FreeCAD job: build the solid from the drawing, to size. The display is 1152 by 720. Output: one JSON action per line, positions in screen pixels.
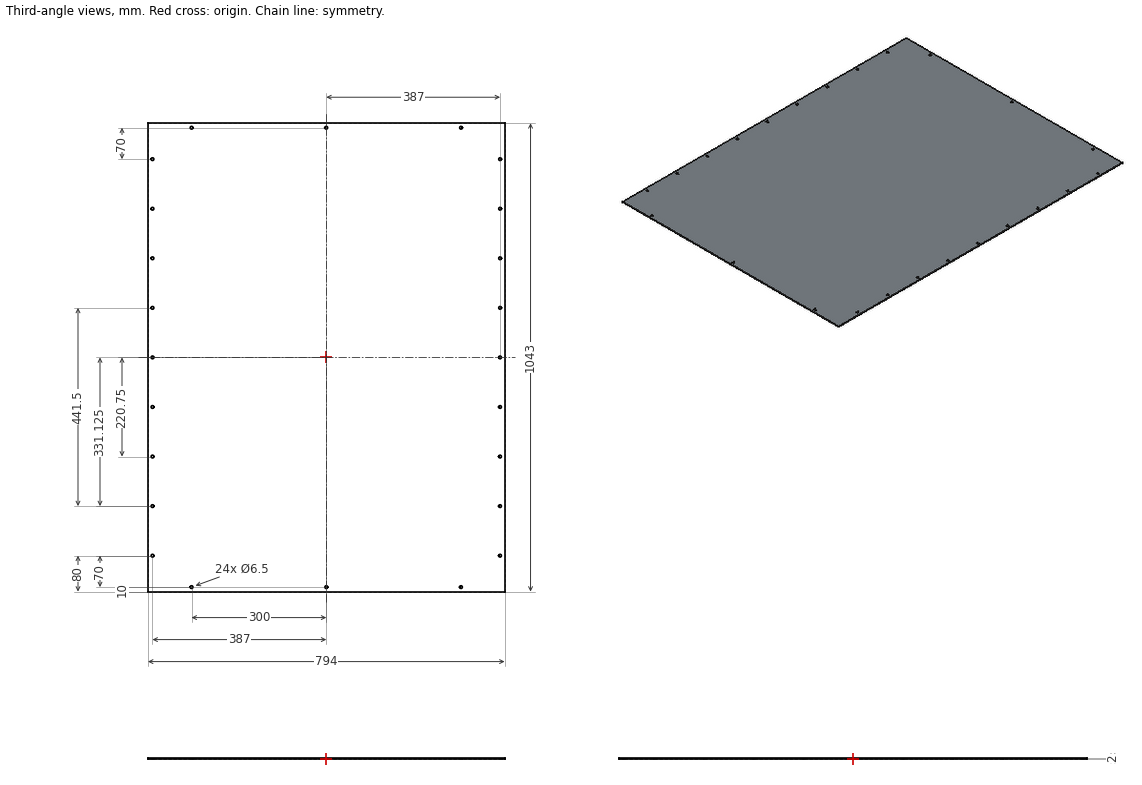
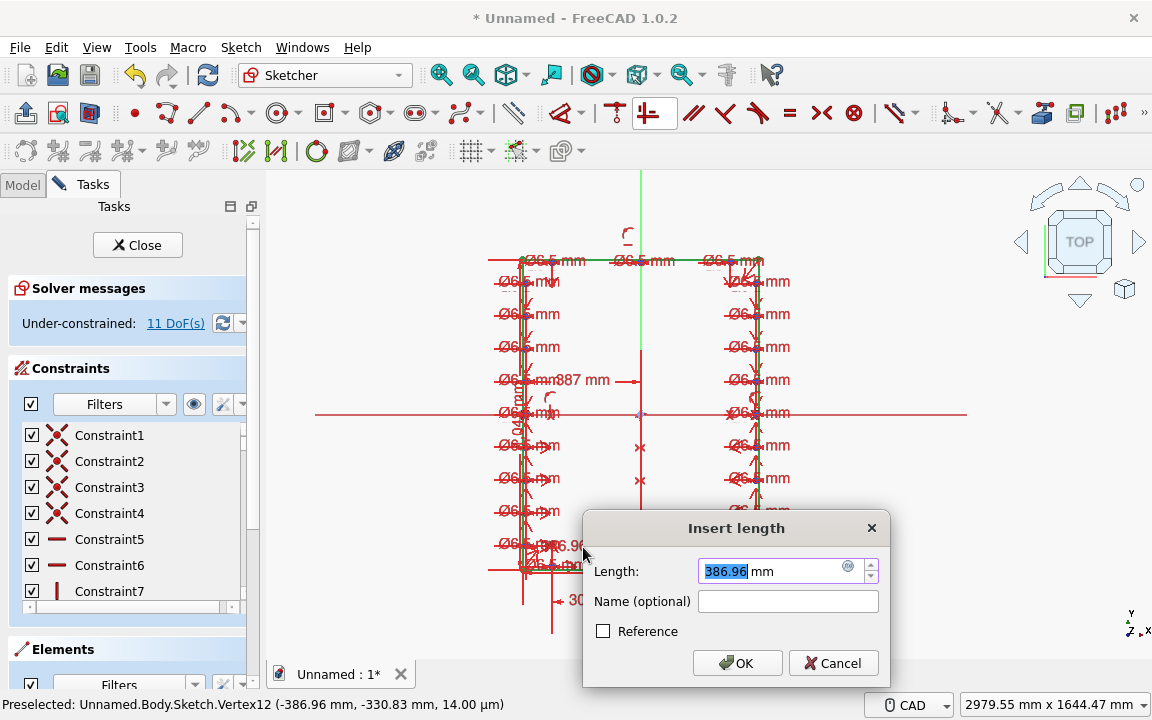
{"action": "type", "text": "387"}
{"action": "key", "text": "Return"}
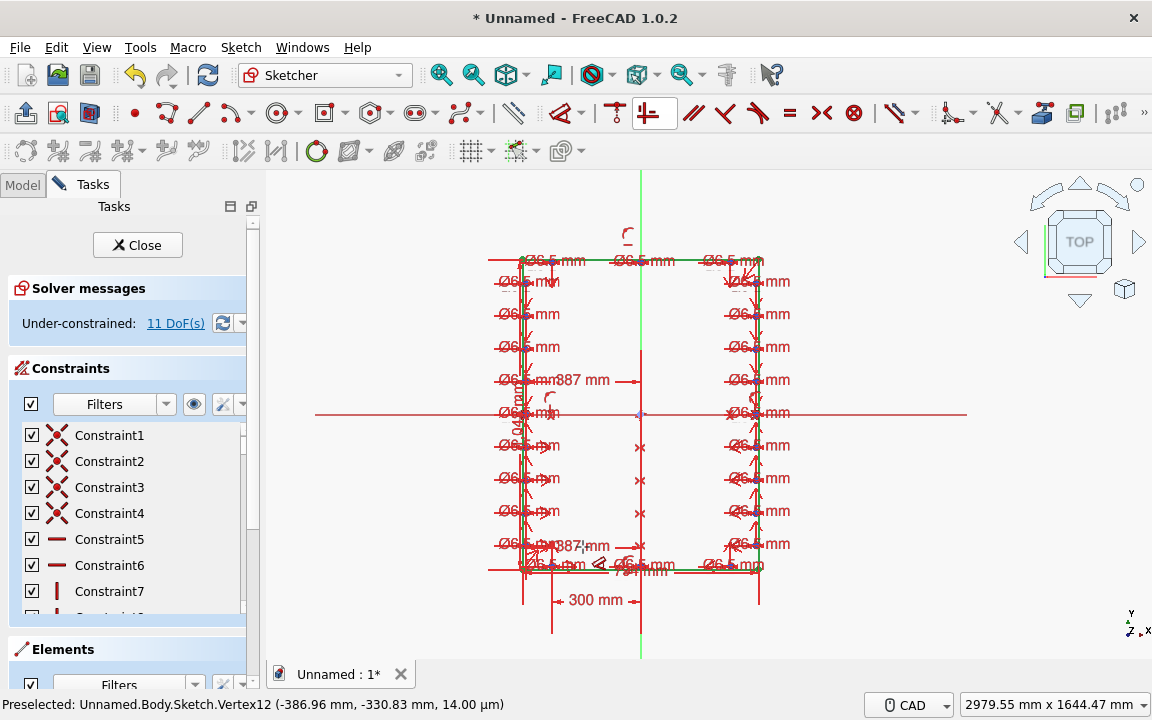
{"action": "left_click", "coordinate": [526, 480]}
{"action": "left_click", "coordinate": [583, 514]}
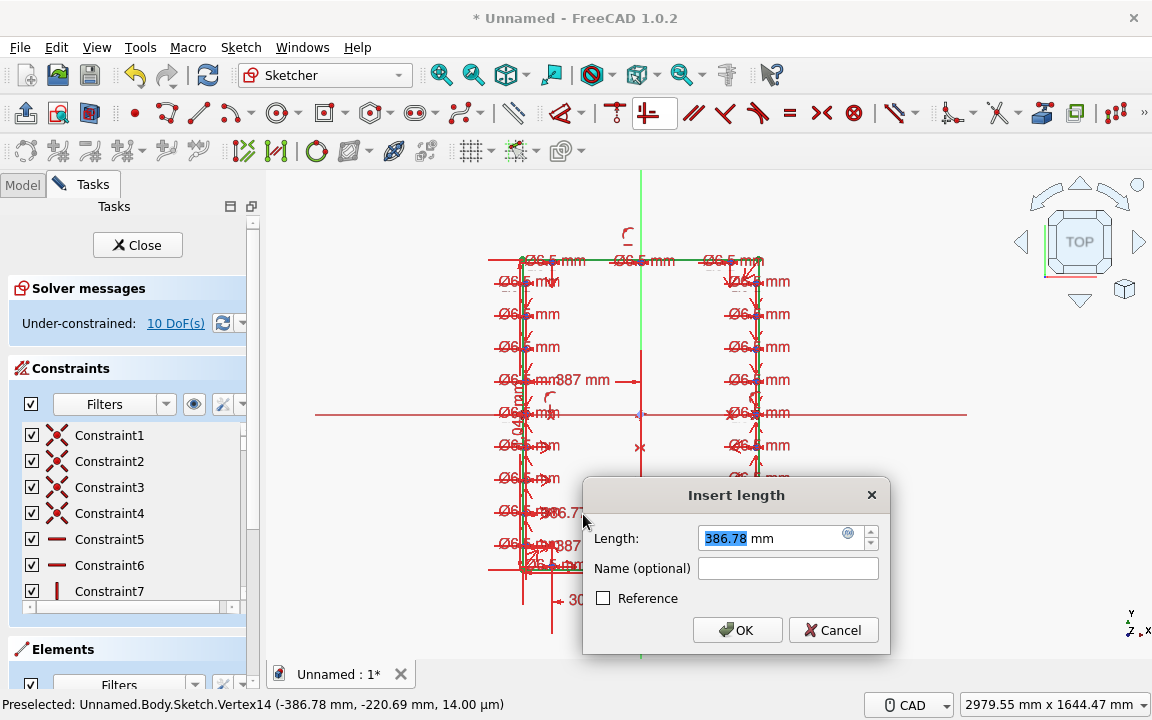
{"action": "type", "text": "387"}
{"action": "key", "text": "Return"}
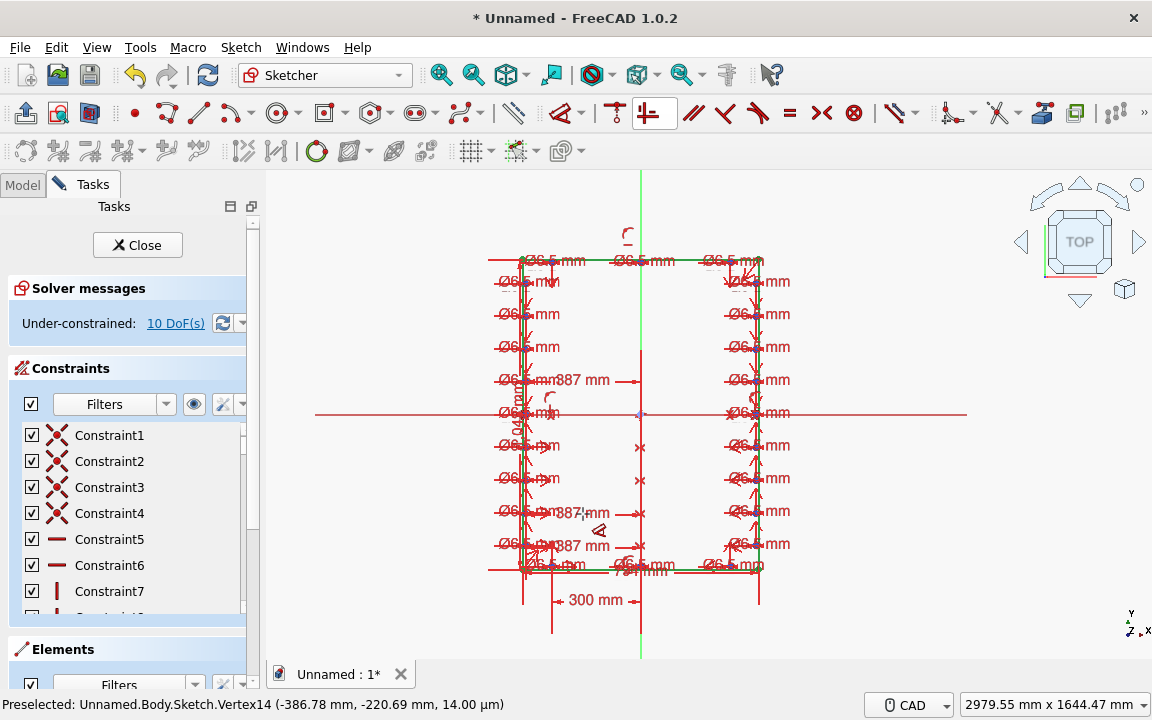
{"action": "left_click", "coordinate": [526, 447]}
{"action": "left_click", "coordinate": [583, 481]}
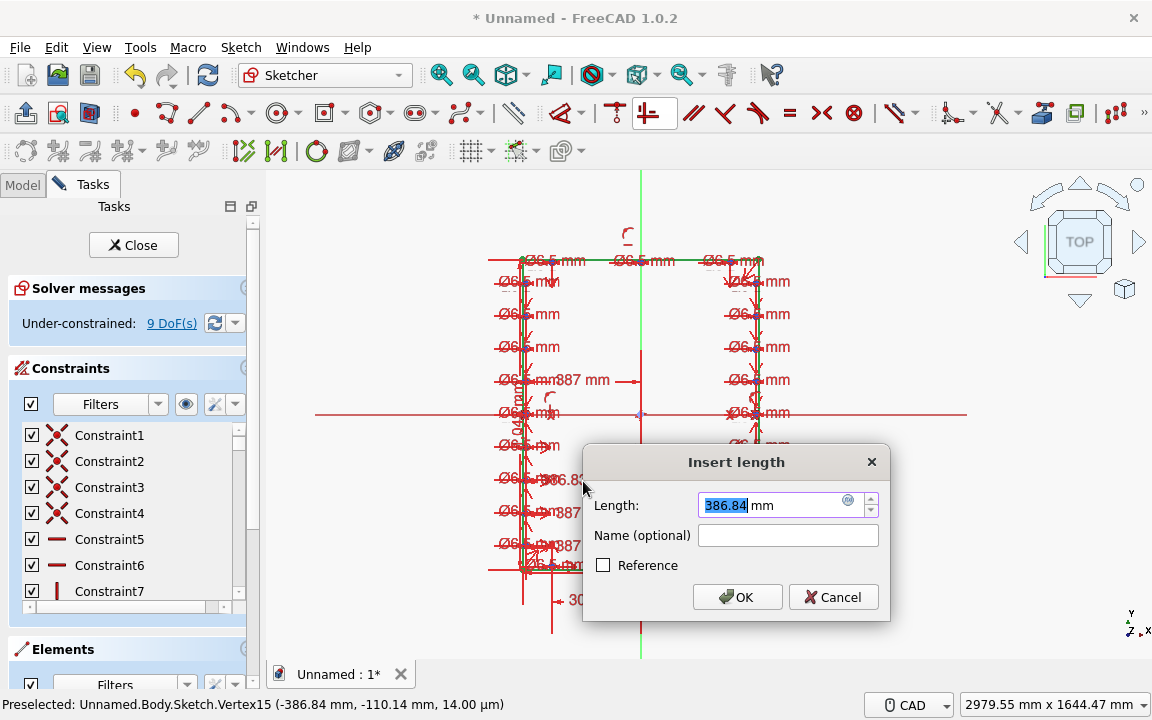
{"action": "type", "text": "387"}
{"action": "key", "text": "Return"}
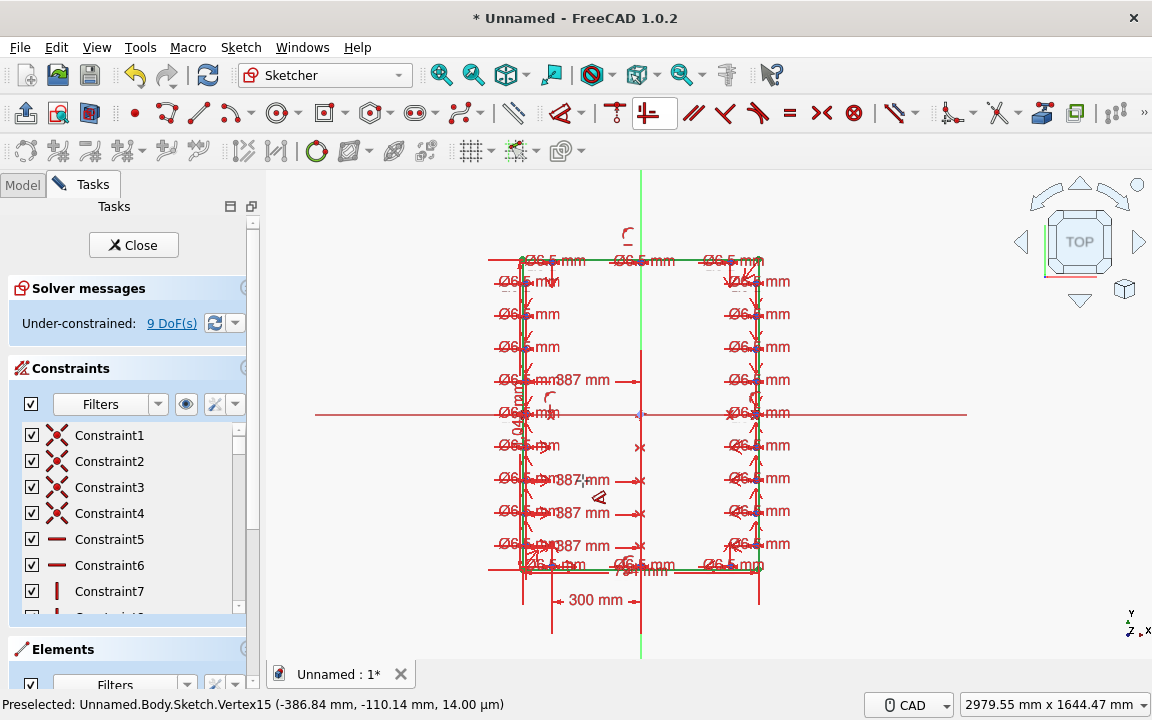
{"action": "left_click", "coordinate": [526, 415]}
{"action": "left_click", "coordinate": [583, 449]}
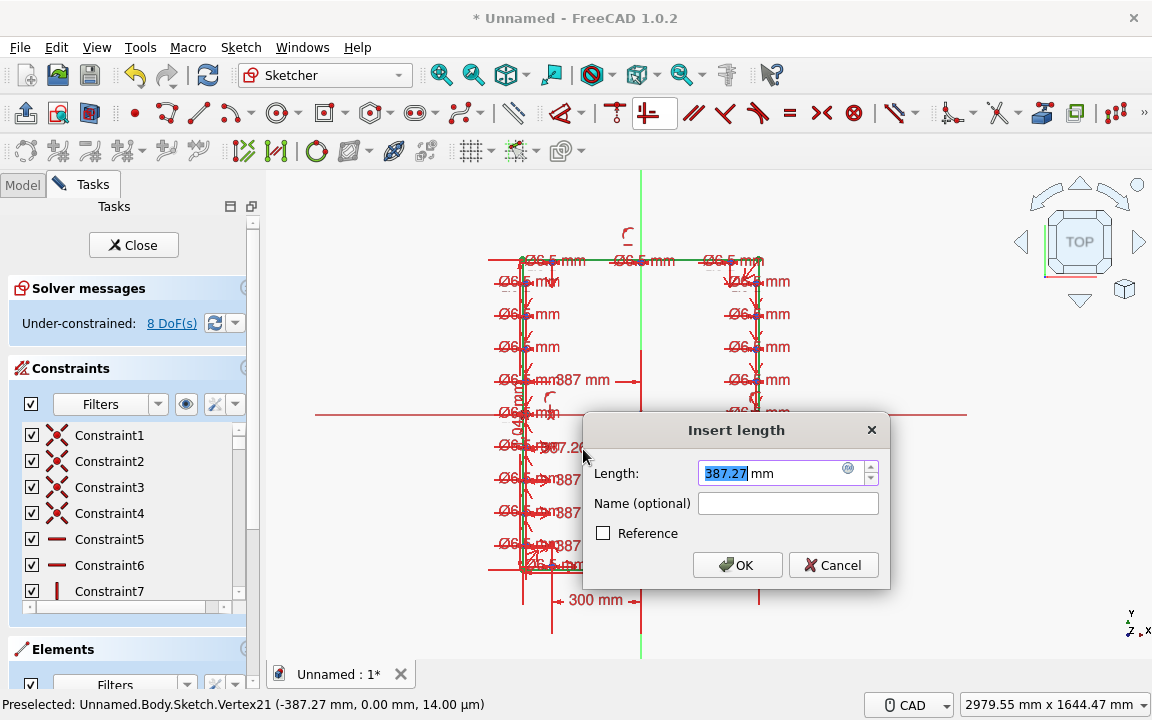
{"action": "type", "text": "387"}
{"action": "key", "text": "Return"}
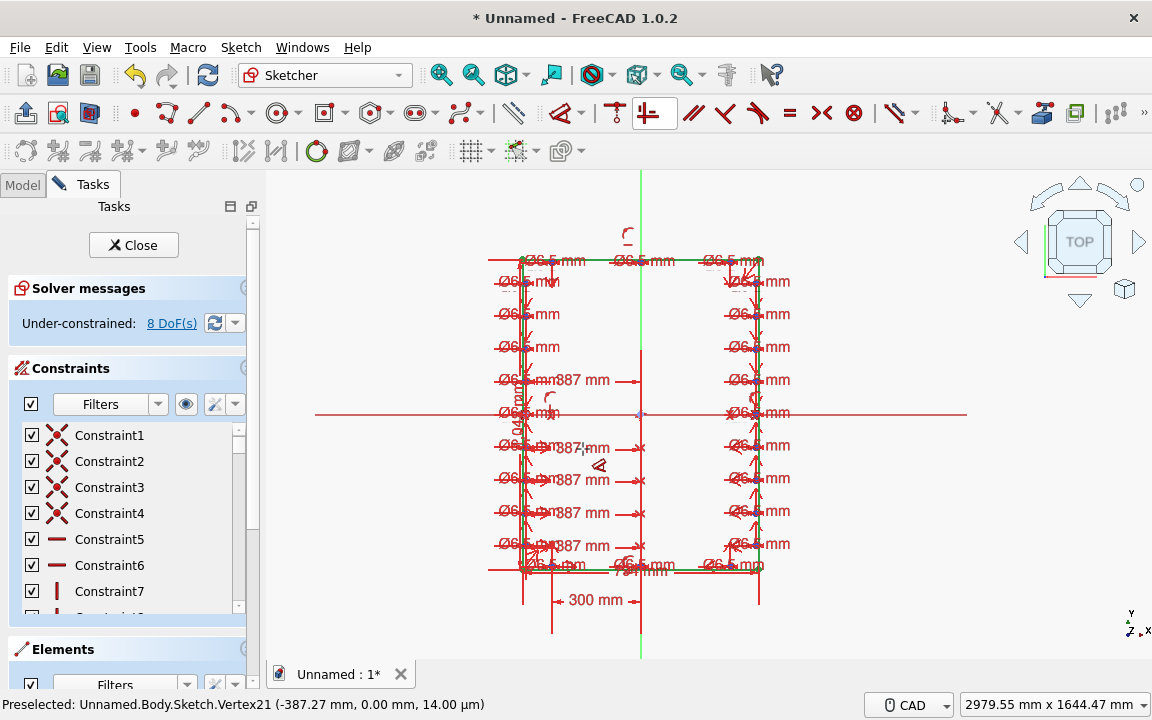
{"action": "left_click", "coordinate": [756, 415]}
{"action": "left_click", "coordinate": [698, 449]}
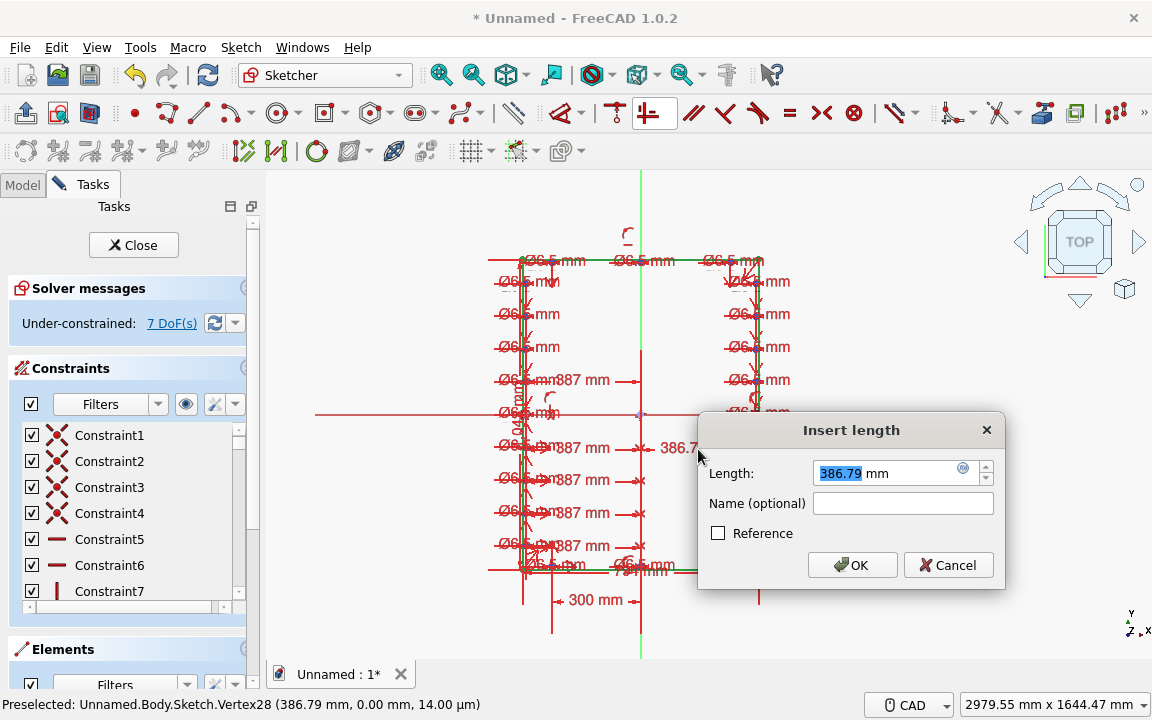
{"action": "type", "text": "387"}
{"action": "key", "text": "Return"}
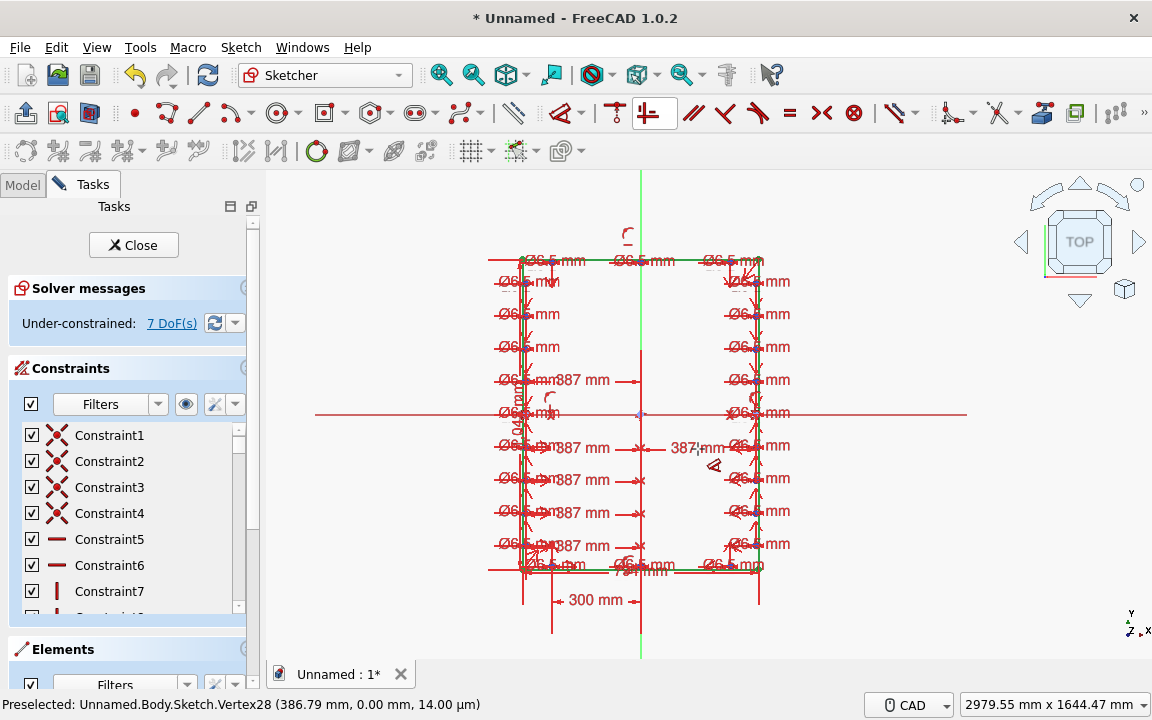
{"action": "scroll", "coordinate": [523, 570], "scroll_direction": "up", "scroll_amount": 13}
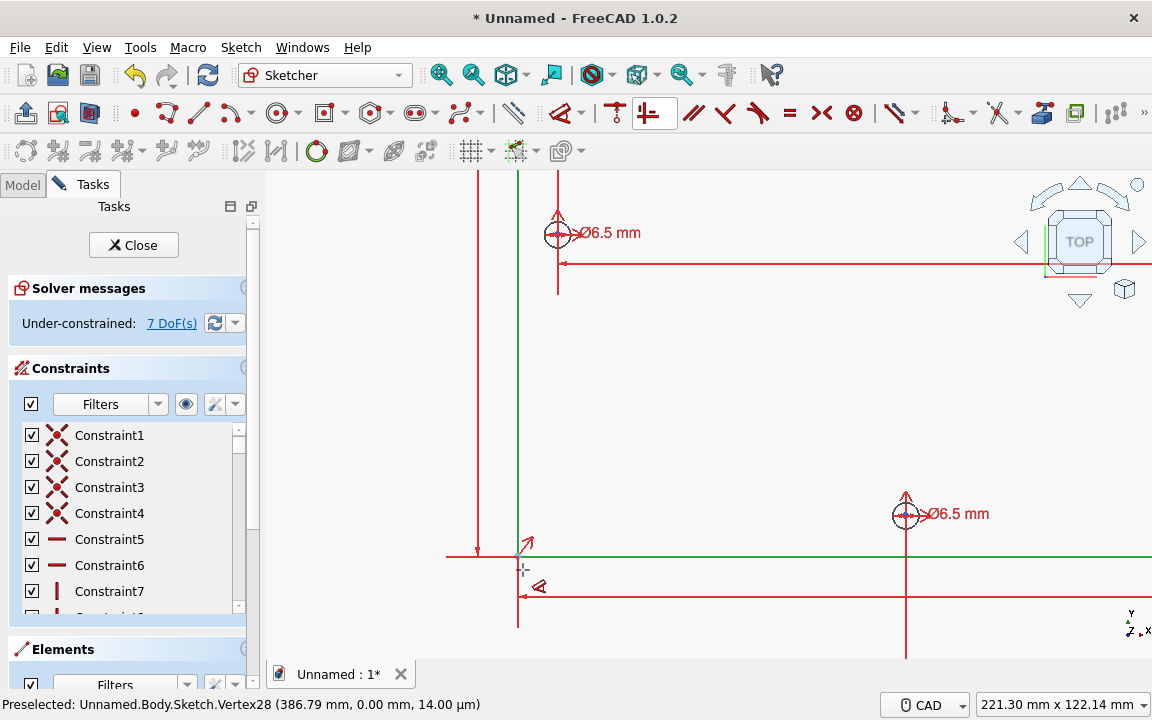
{"action": "left_click", "coordinate": [518, 557]}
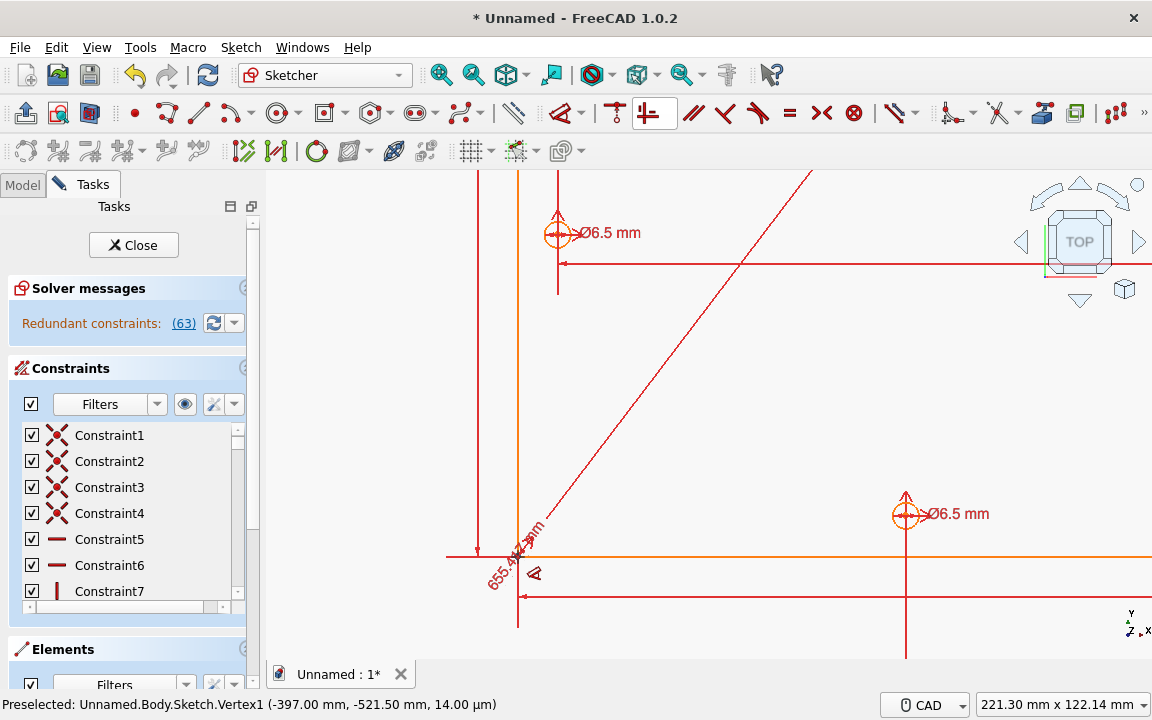
{"action": "left_click", "coordinate": [906, 516]}
{"action": "left_click", "coordinate": [484, 536]}